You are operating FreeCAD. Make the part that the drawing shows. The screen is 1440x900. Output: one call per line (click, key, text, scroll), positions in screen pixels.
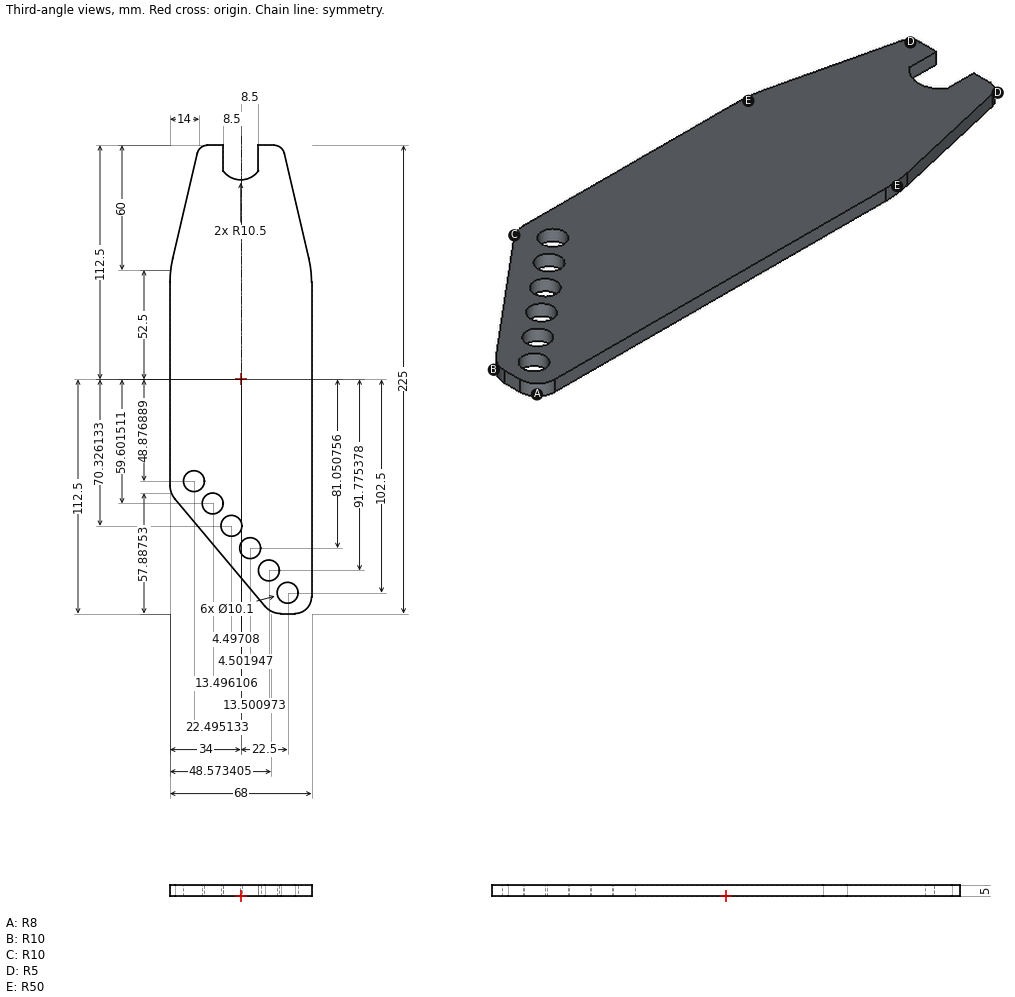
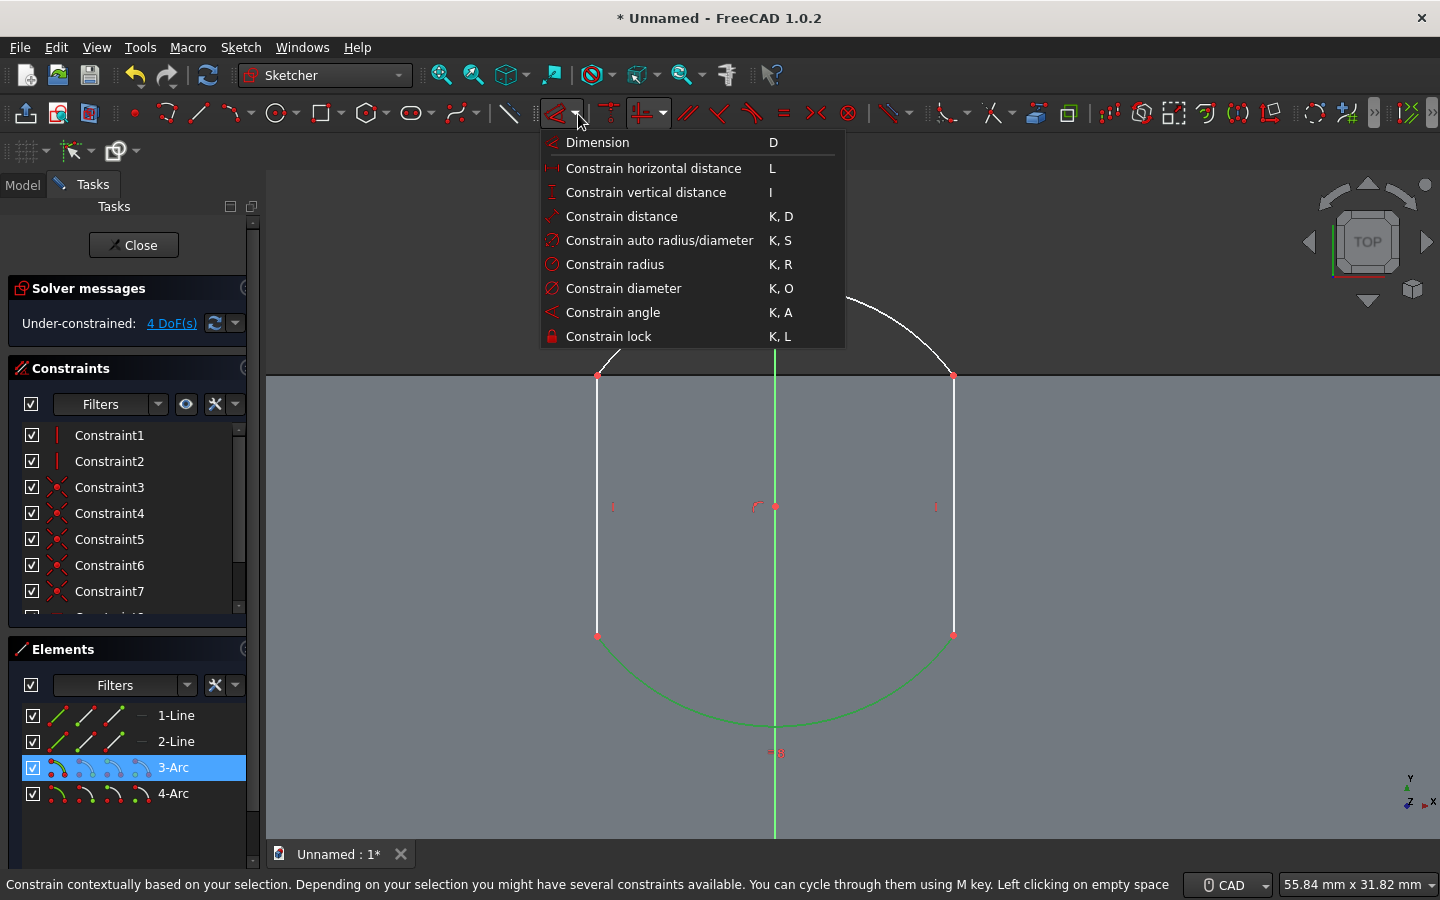
click(693, 264)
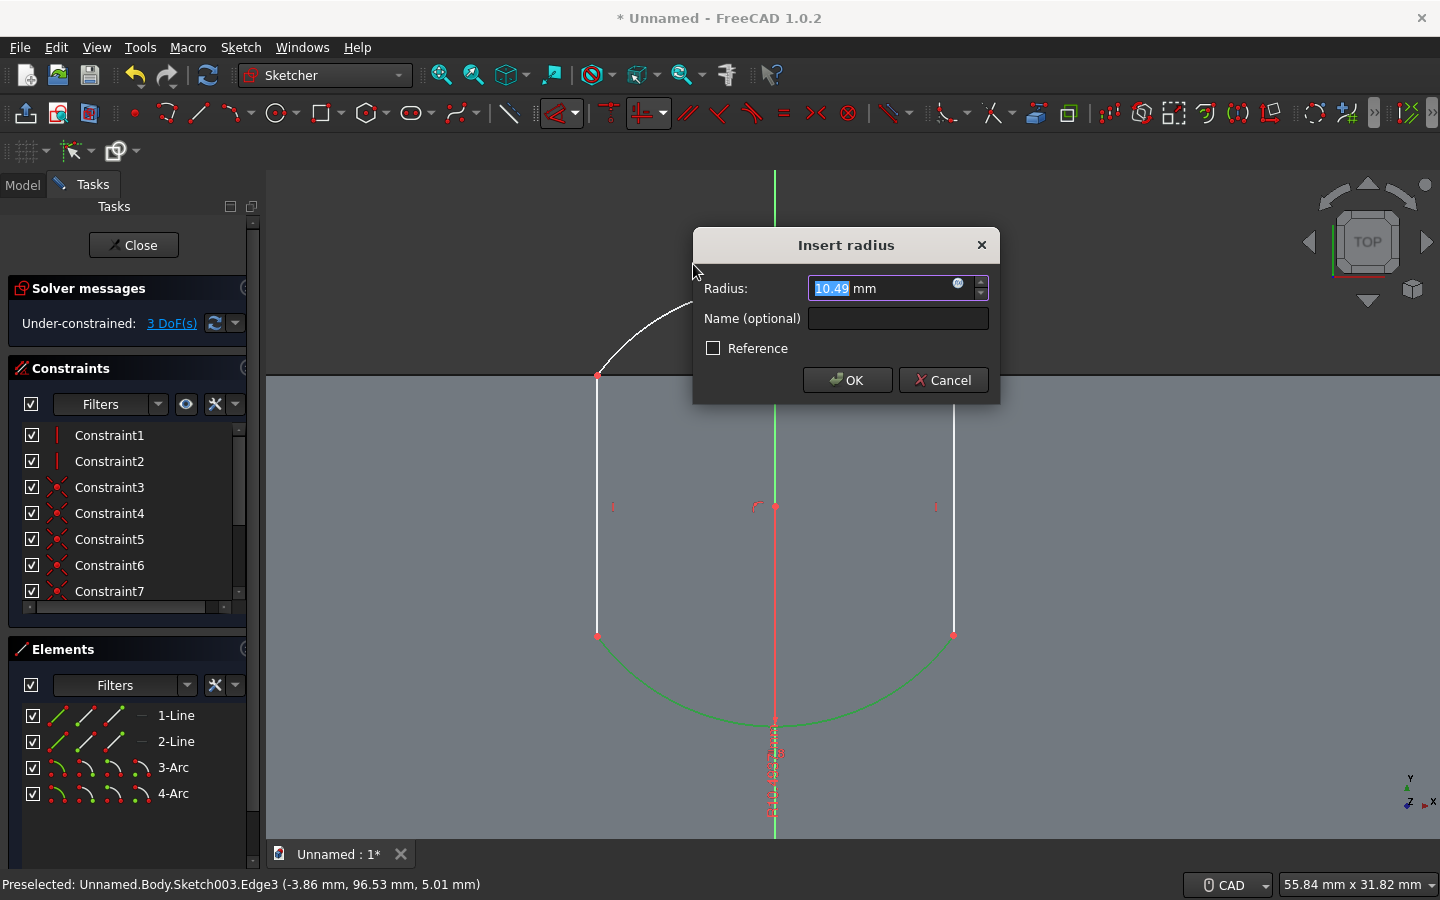
text(10.5)
key(Return)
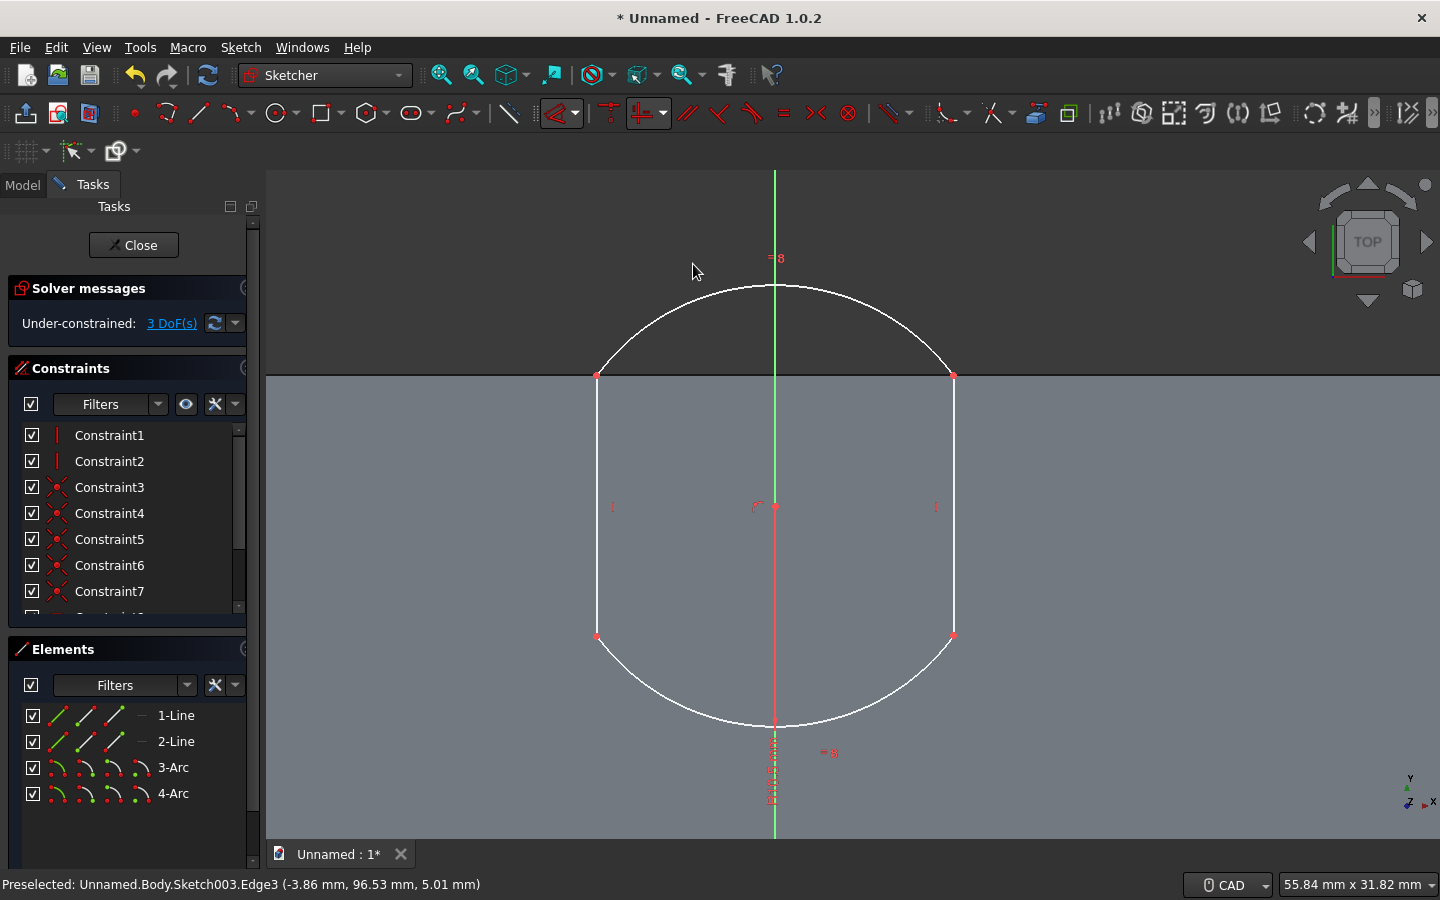
click(597, 376)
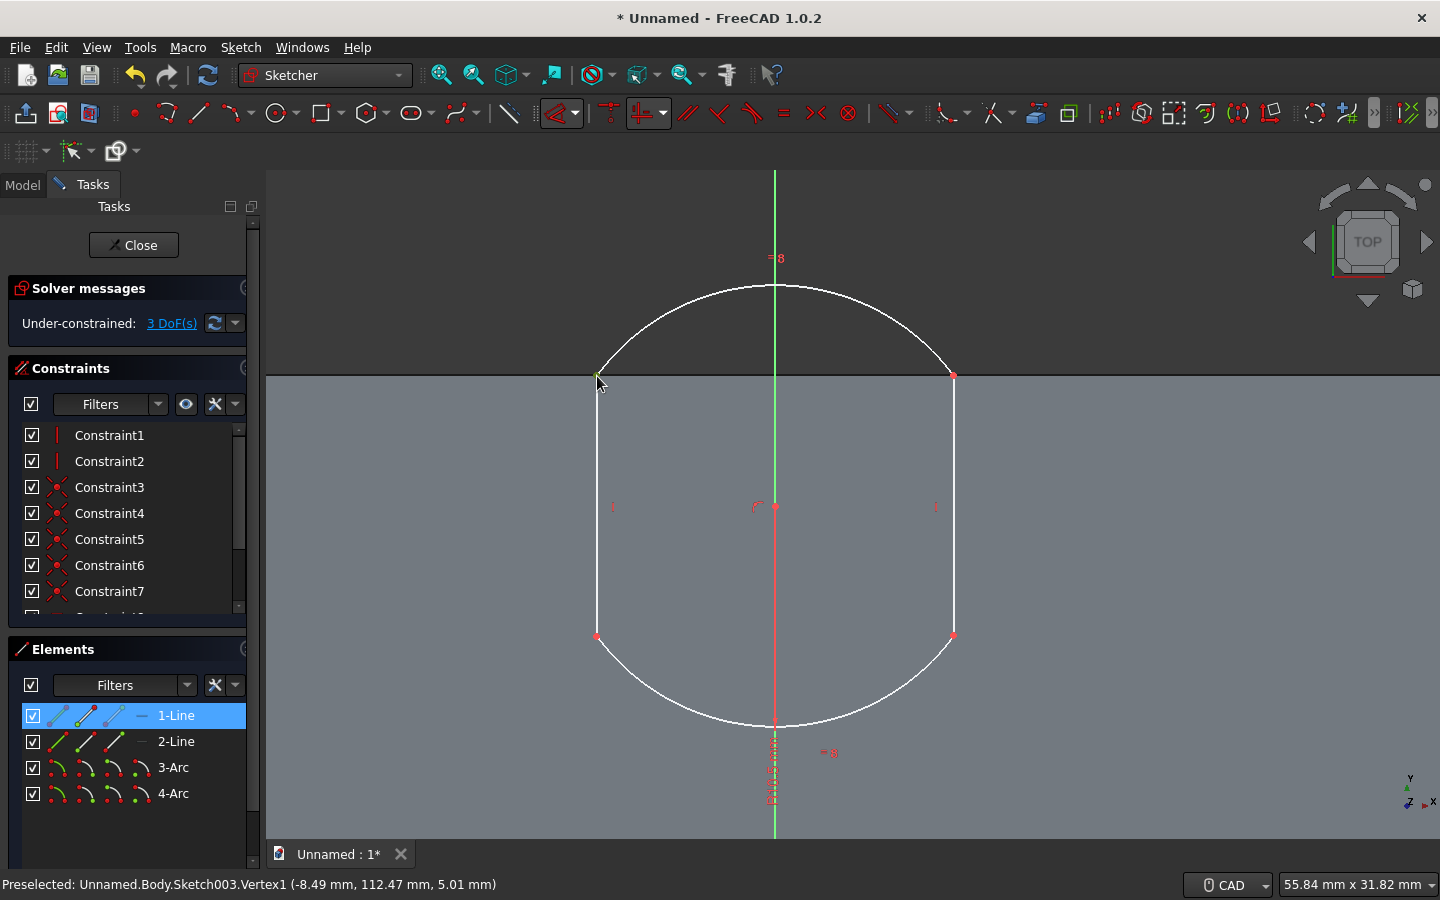
key(l)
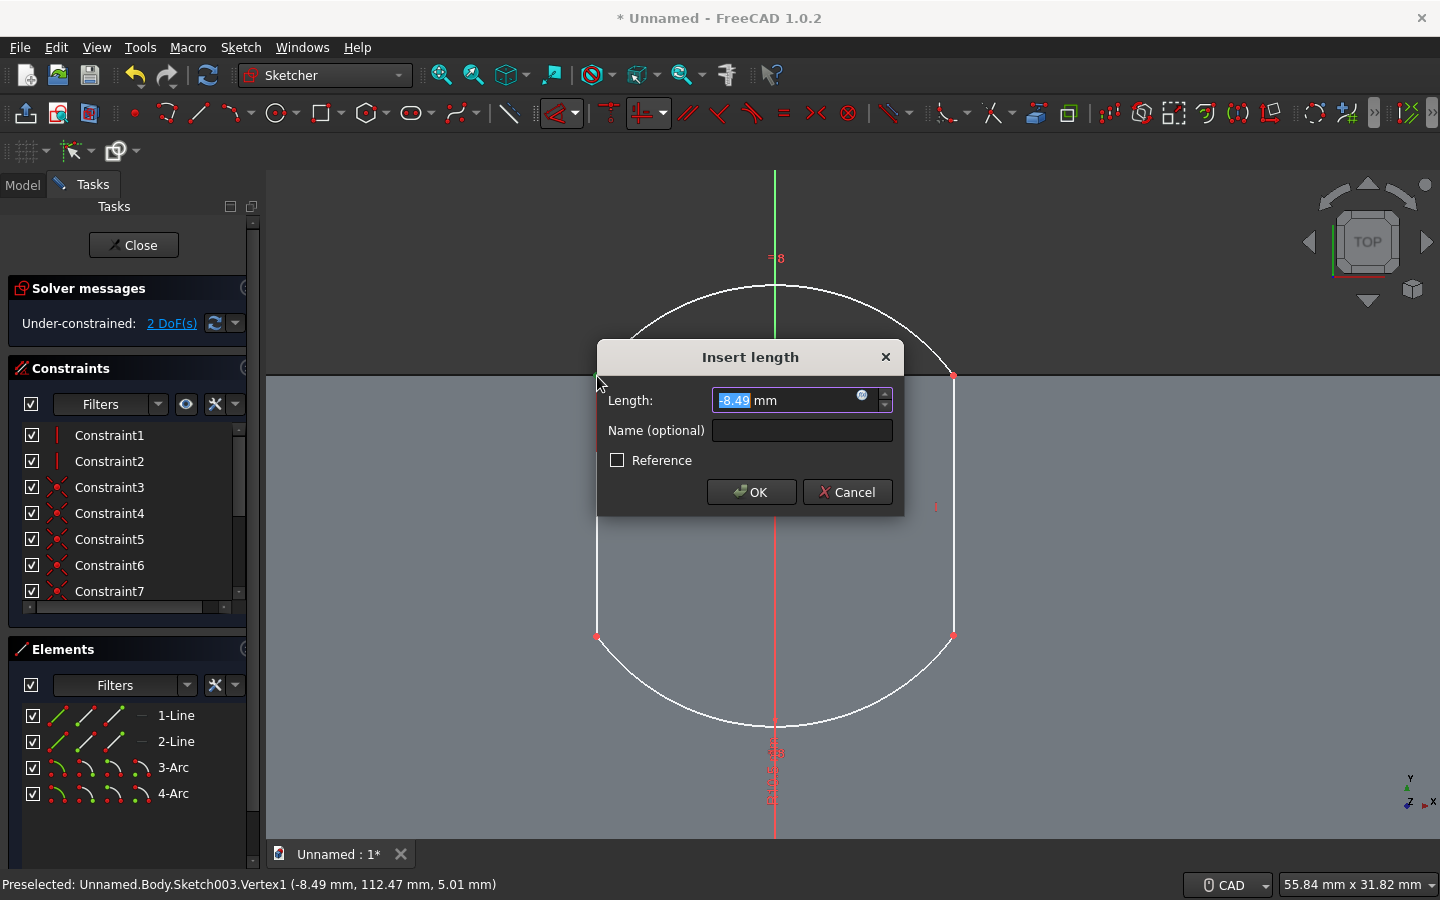
text(-8.5)
key(Return)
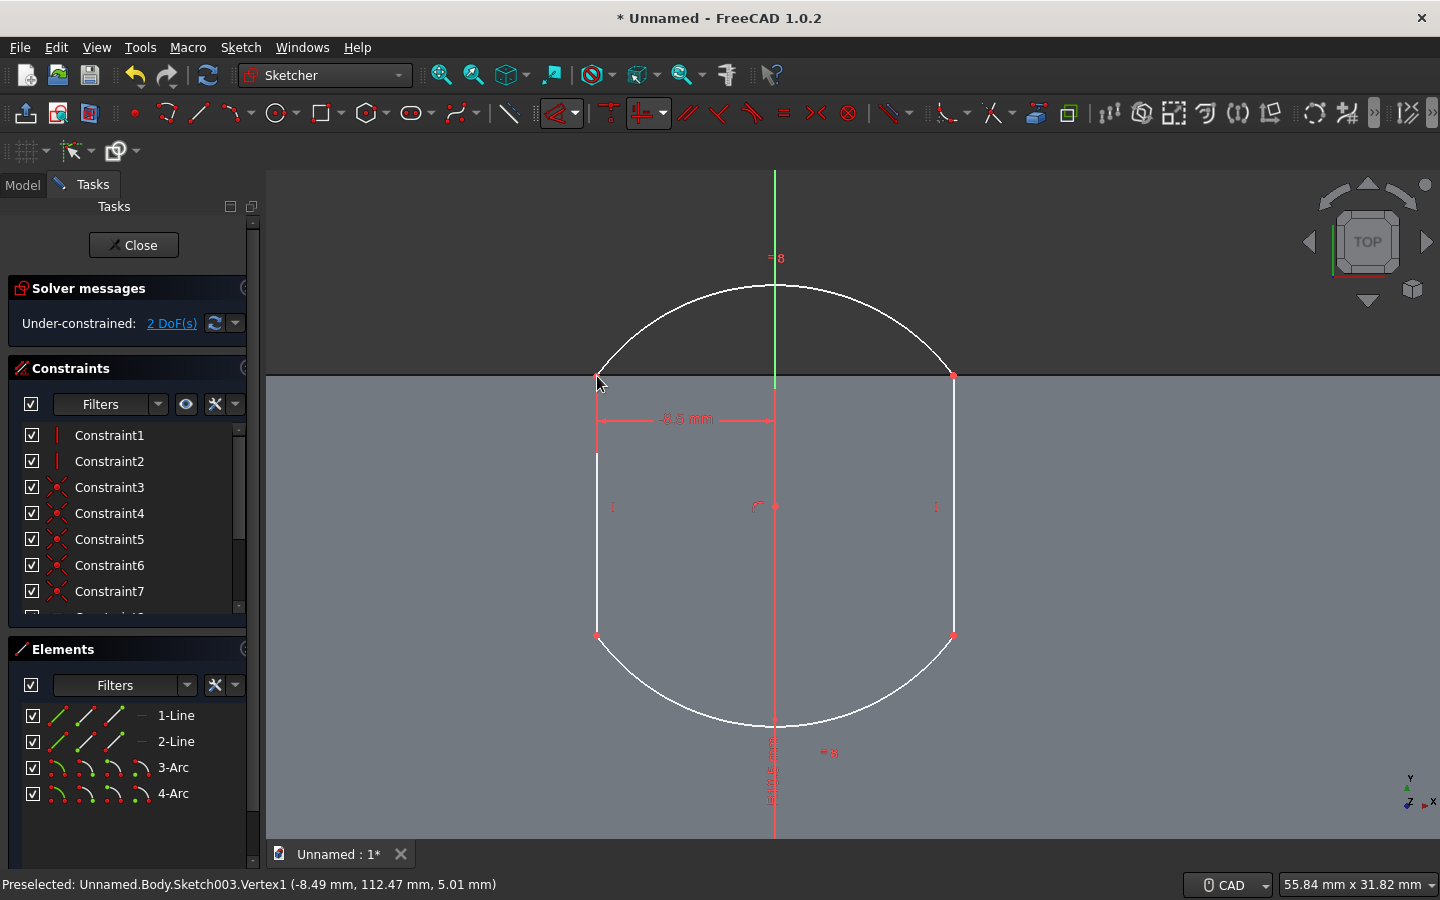
click(954, 636)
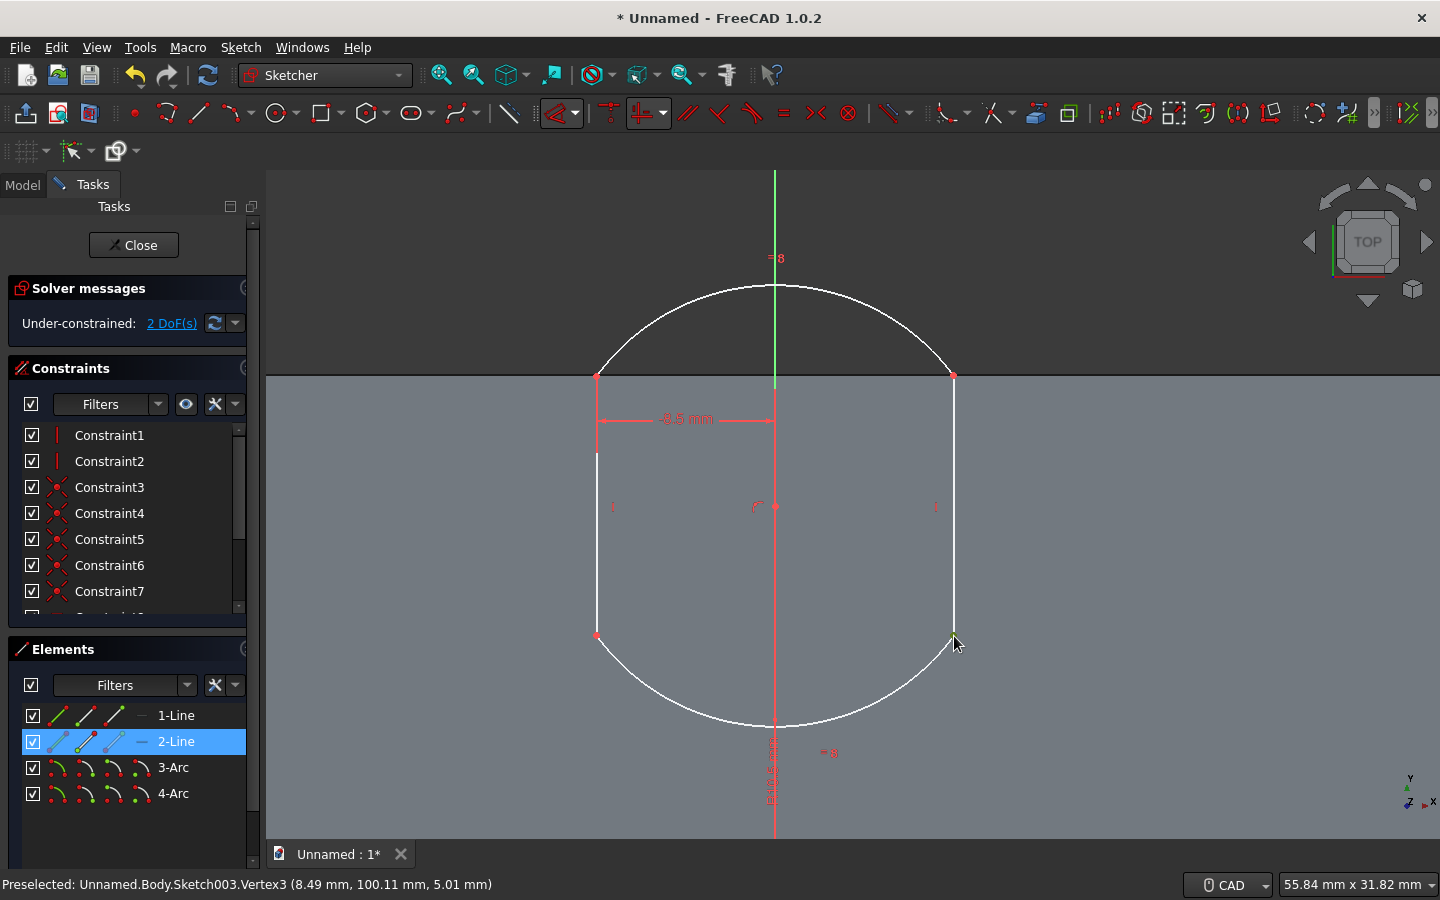
key(l)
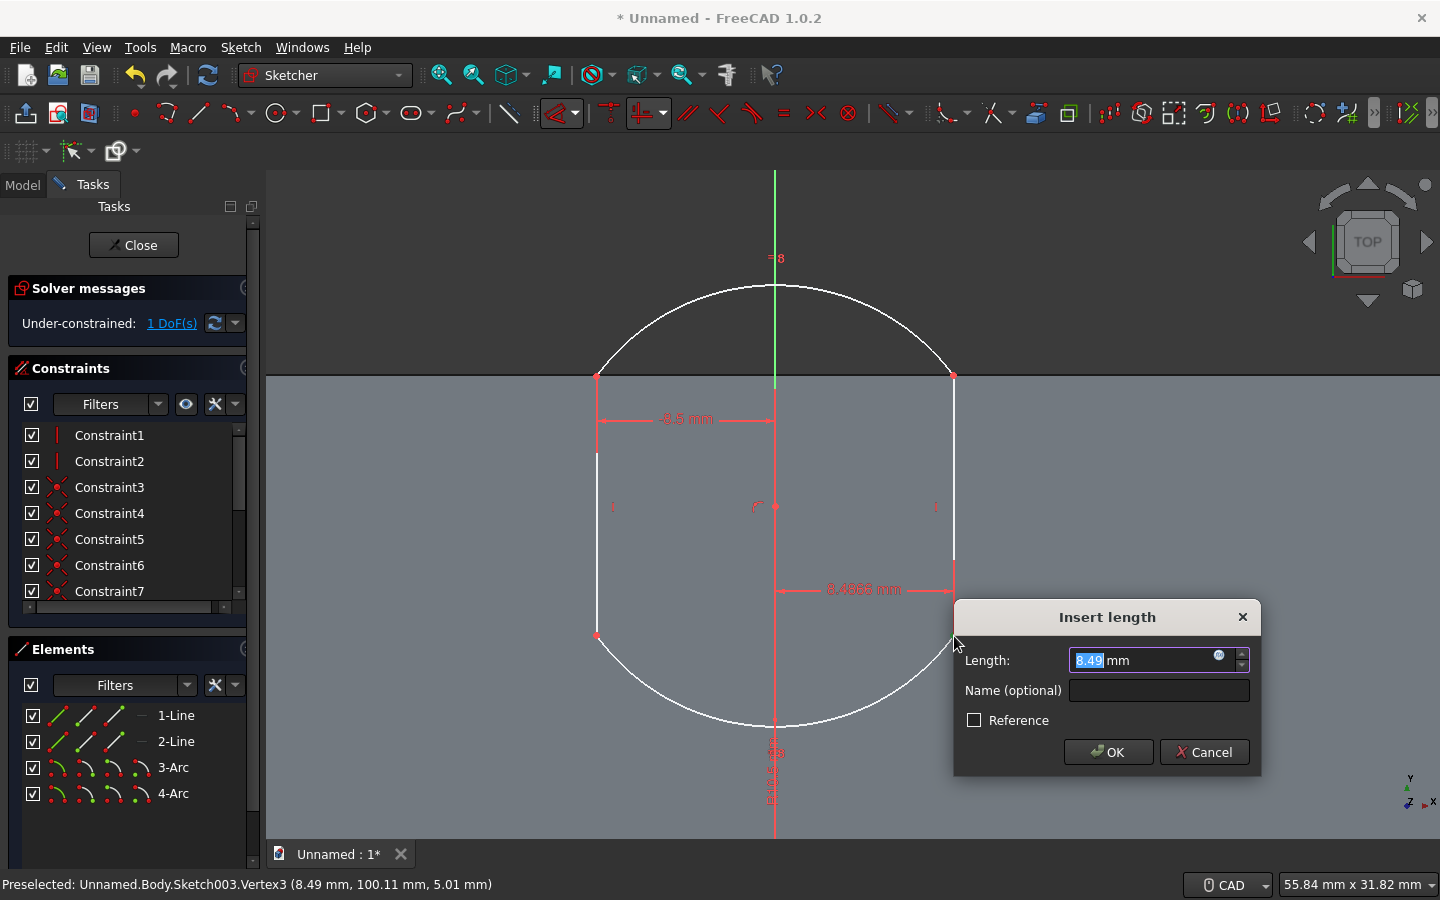
text(8.5)
key(Return)